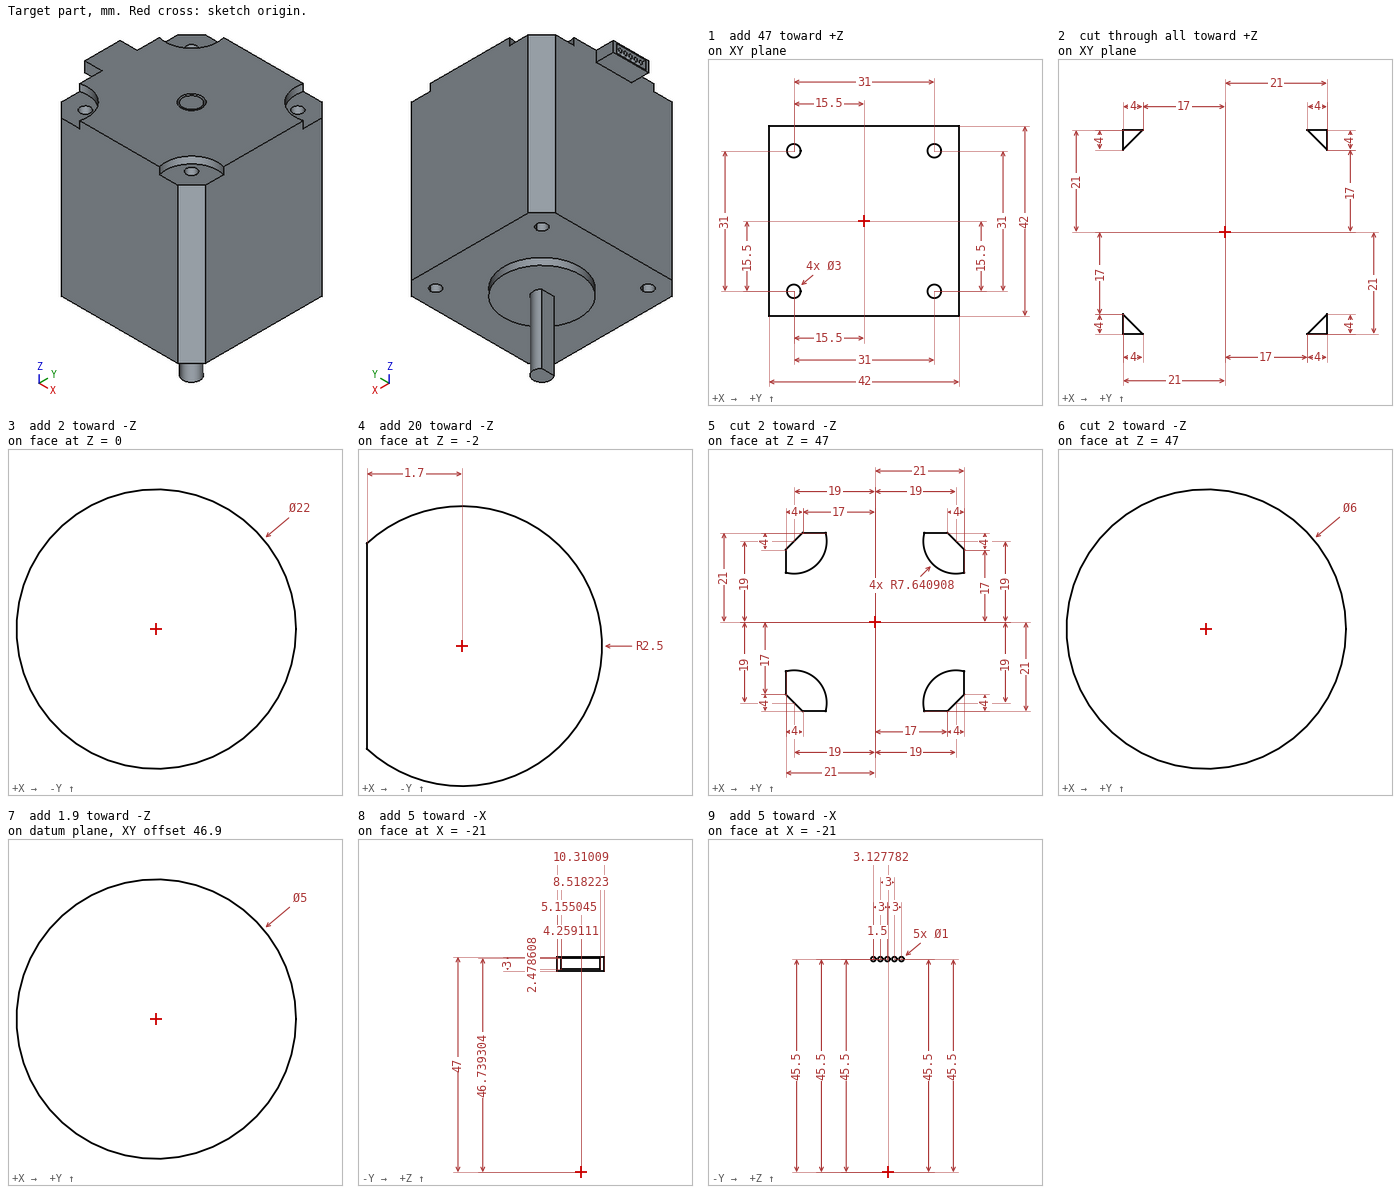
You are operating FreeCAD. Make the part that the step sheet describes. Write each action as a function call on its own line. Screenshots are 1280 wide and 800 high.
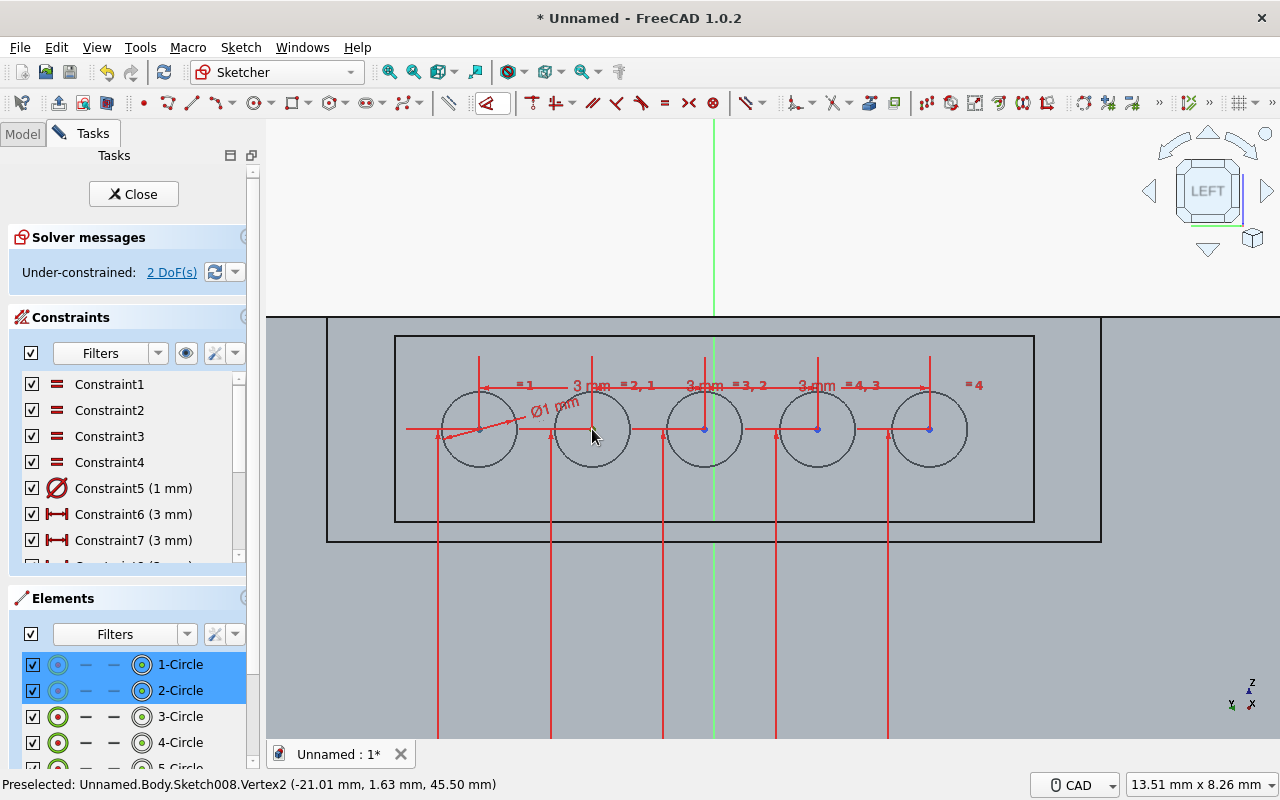
key(l)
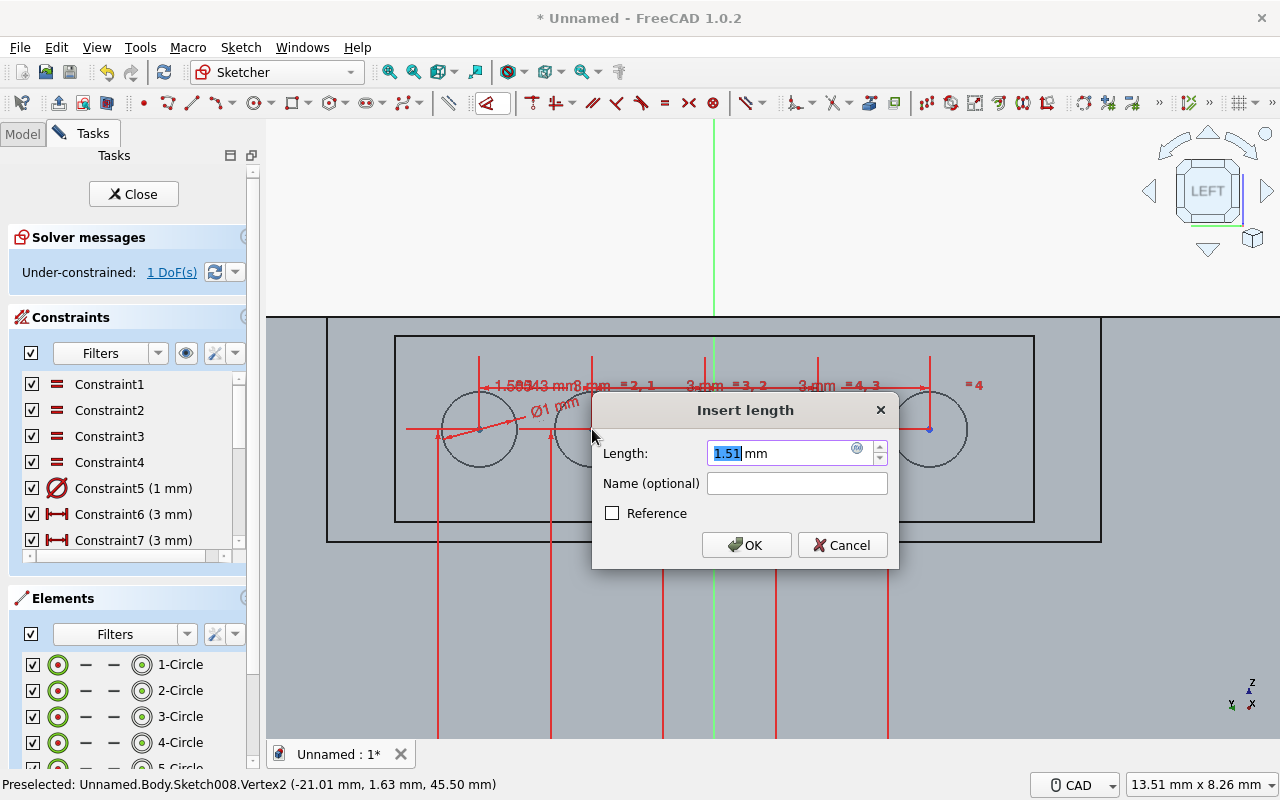
text(1.5)
key(Return)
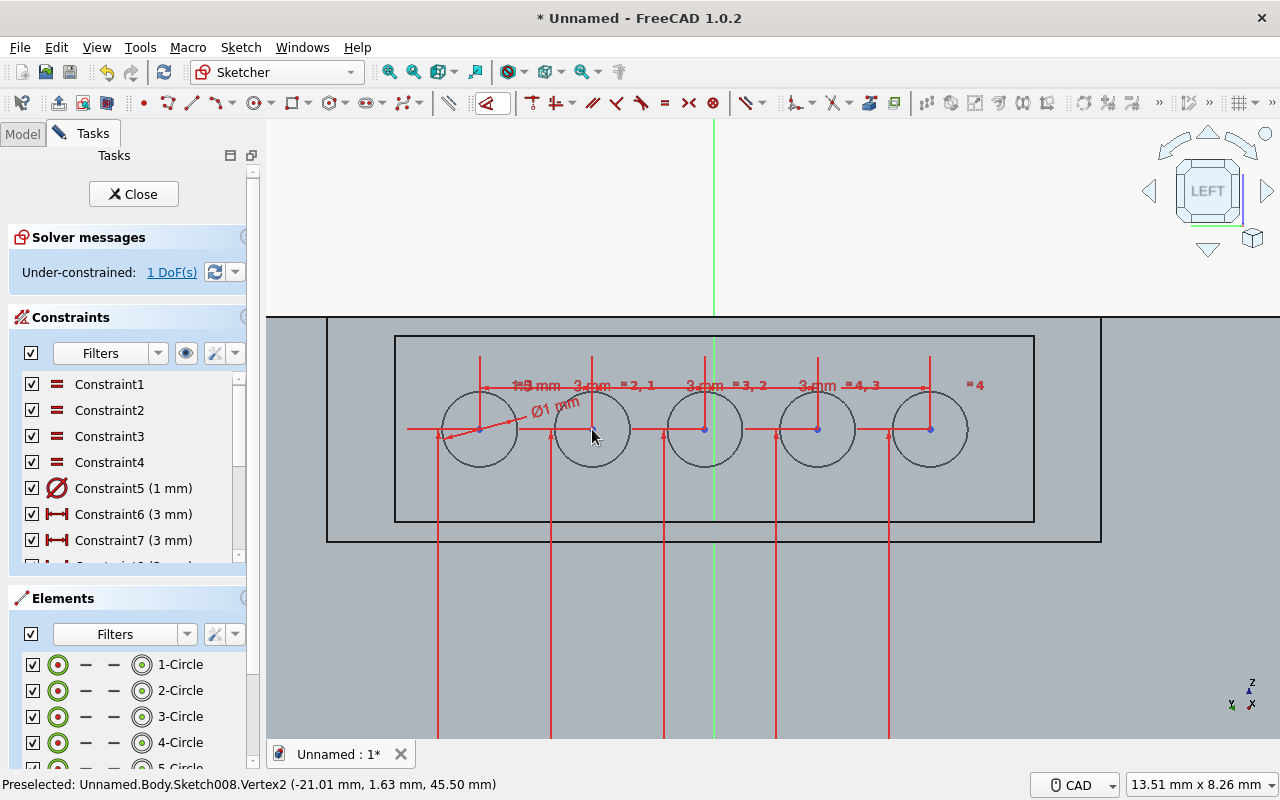
click(480, 429)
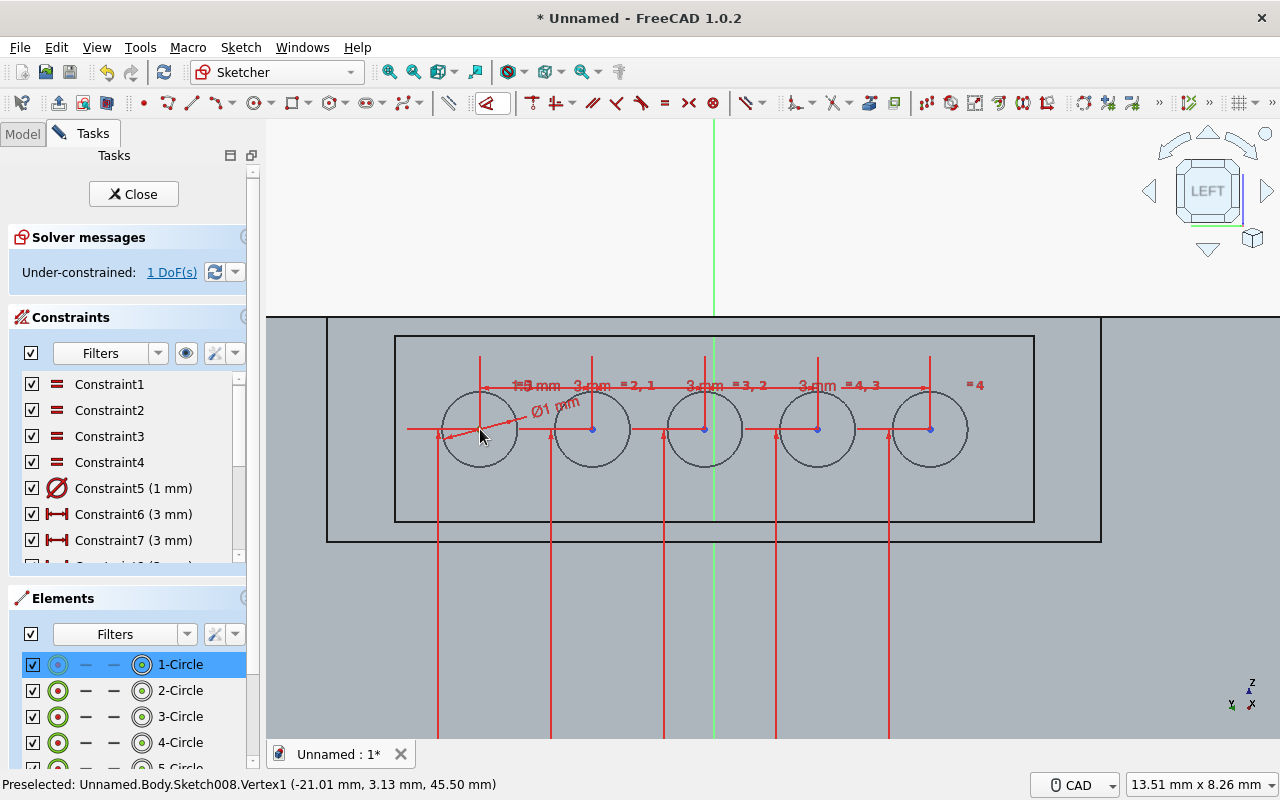
click(504, 104)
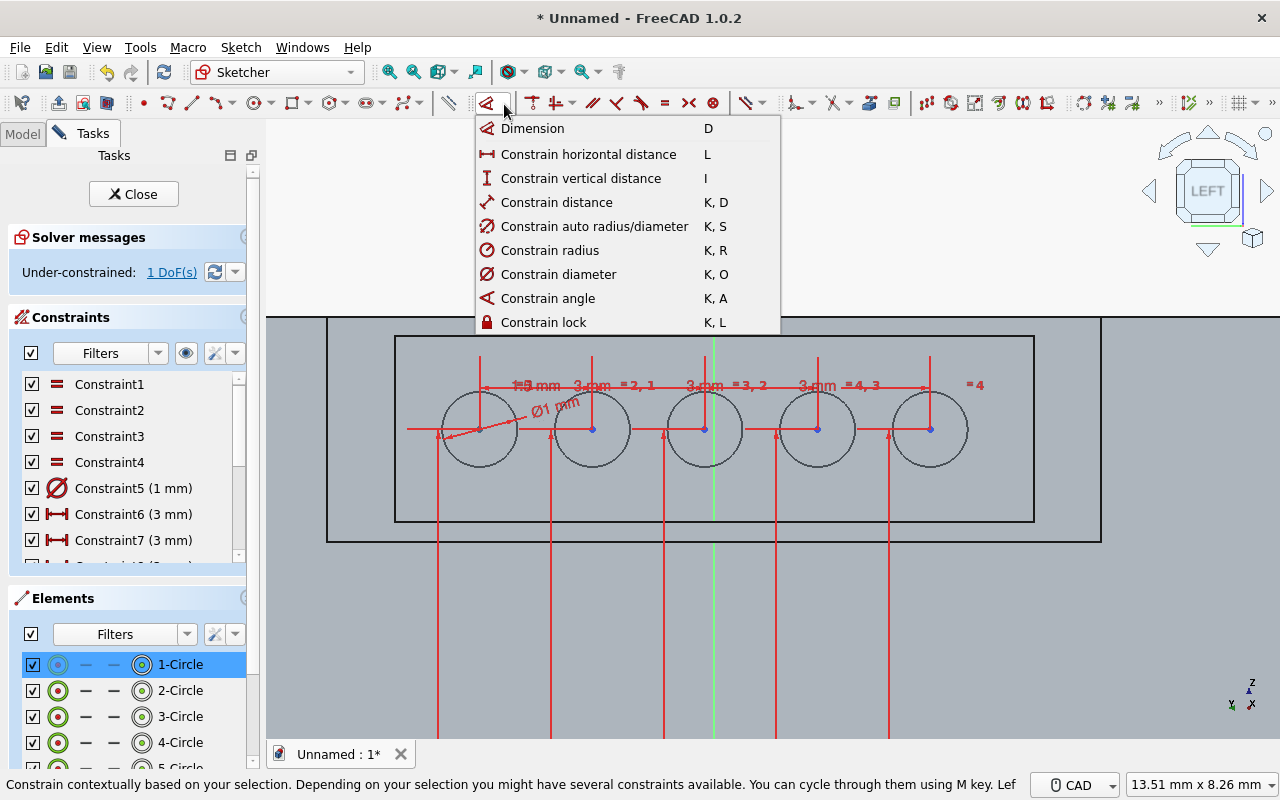
click(628, 154)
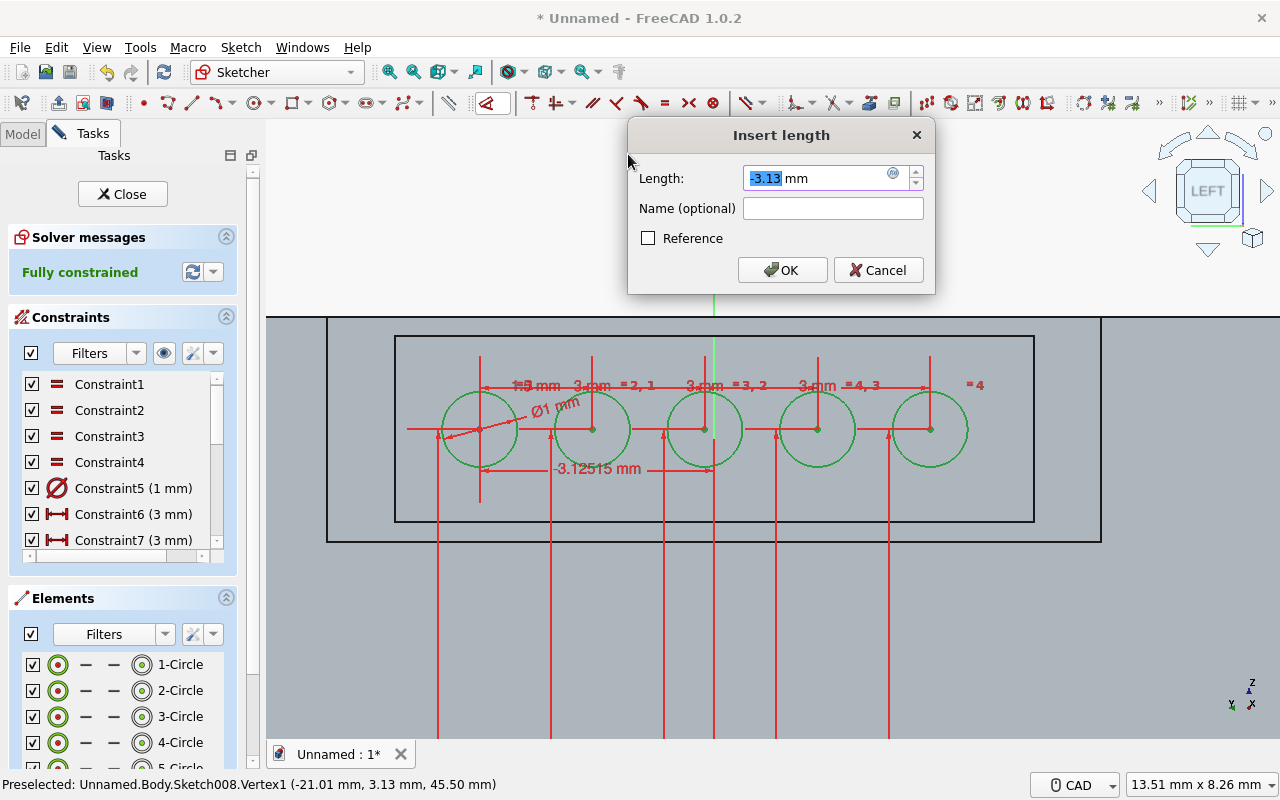
text(-3.127782)
key(Return)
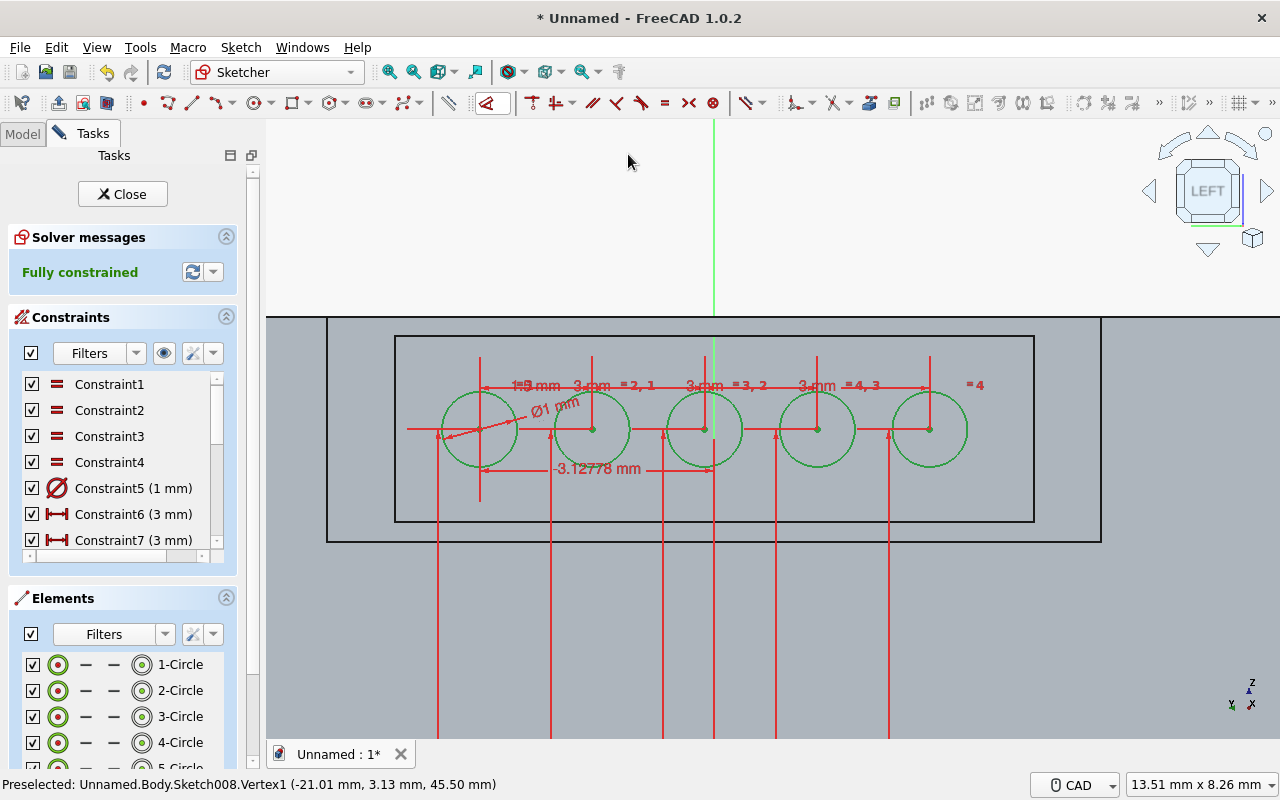
click(123, 194)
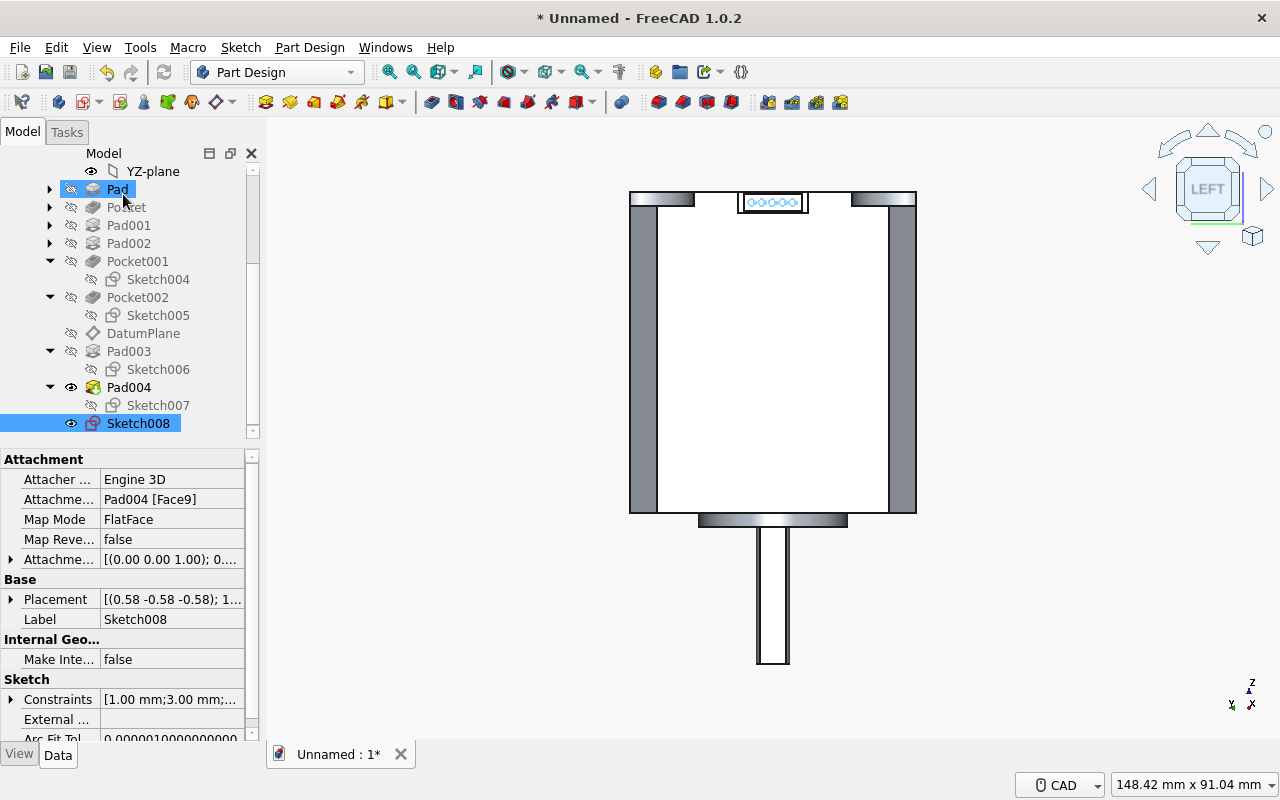
click(266, 102)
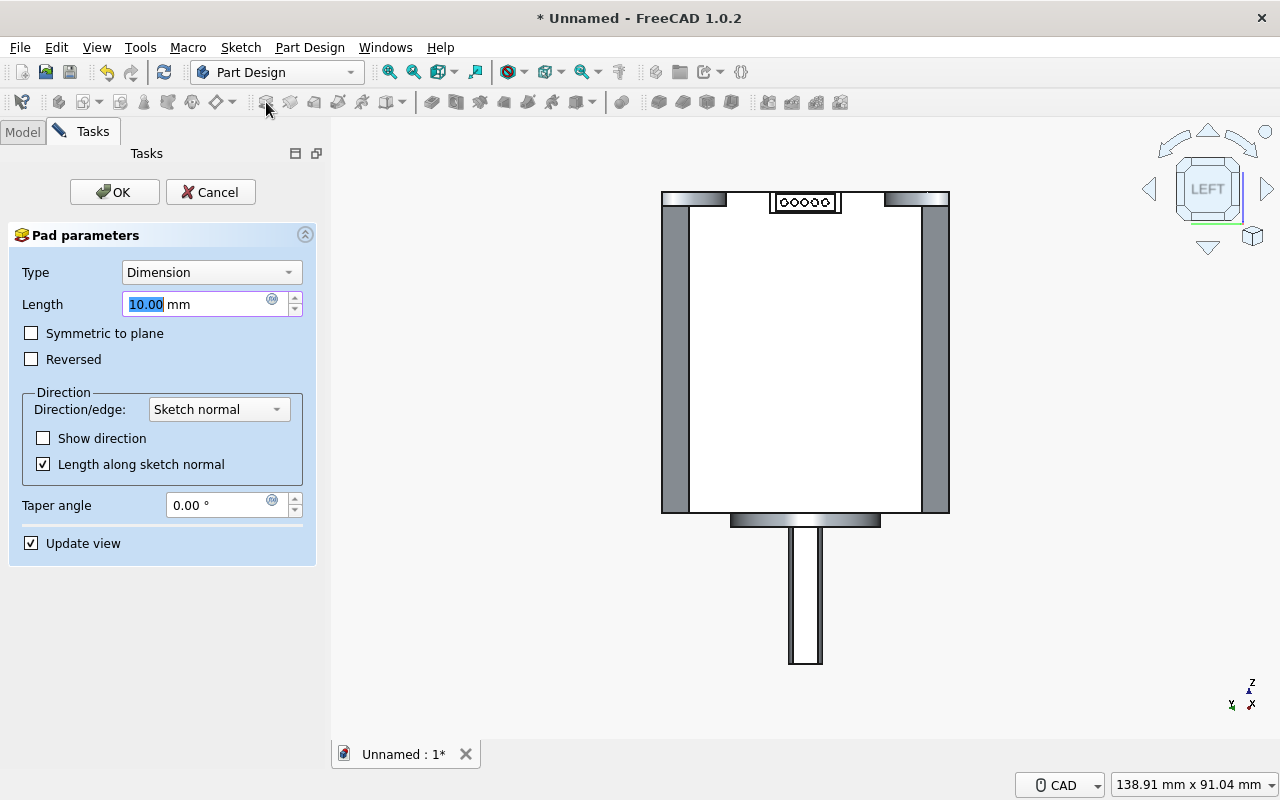
text(5)
key(Tab)